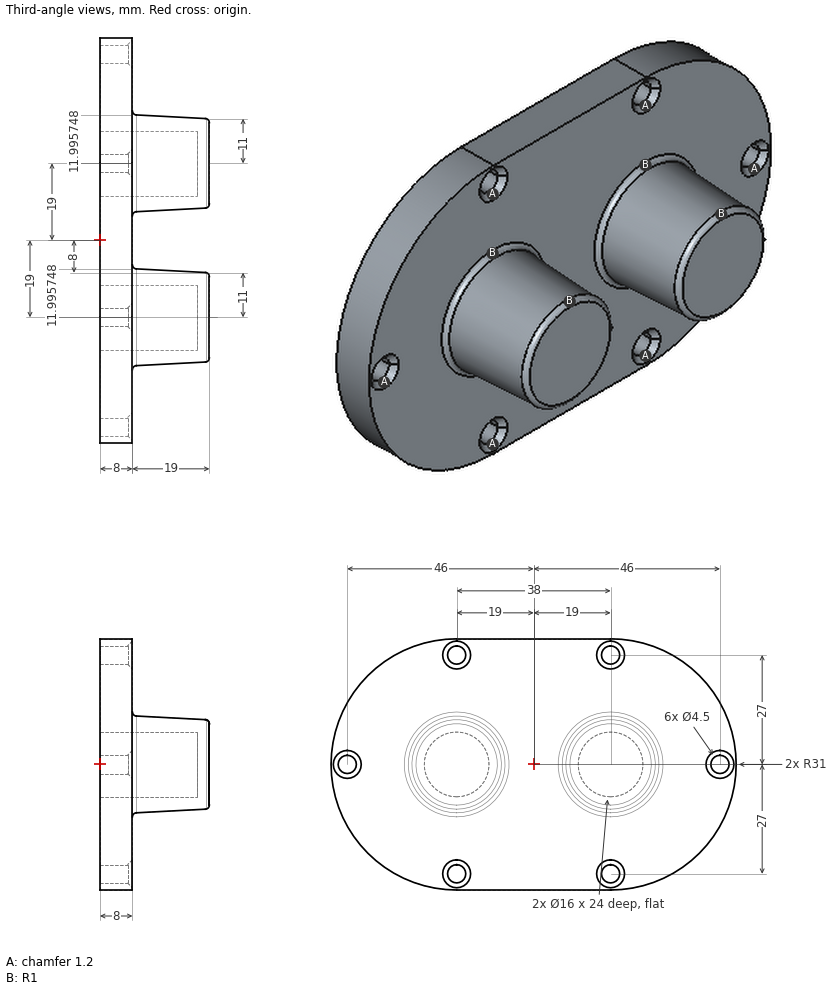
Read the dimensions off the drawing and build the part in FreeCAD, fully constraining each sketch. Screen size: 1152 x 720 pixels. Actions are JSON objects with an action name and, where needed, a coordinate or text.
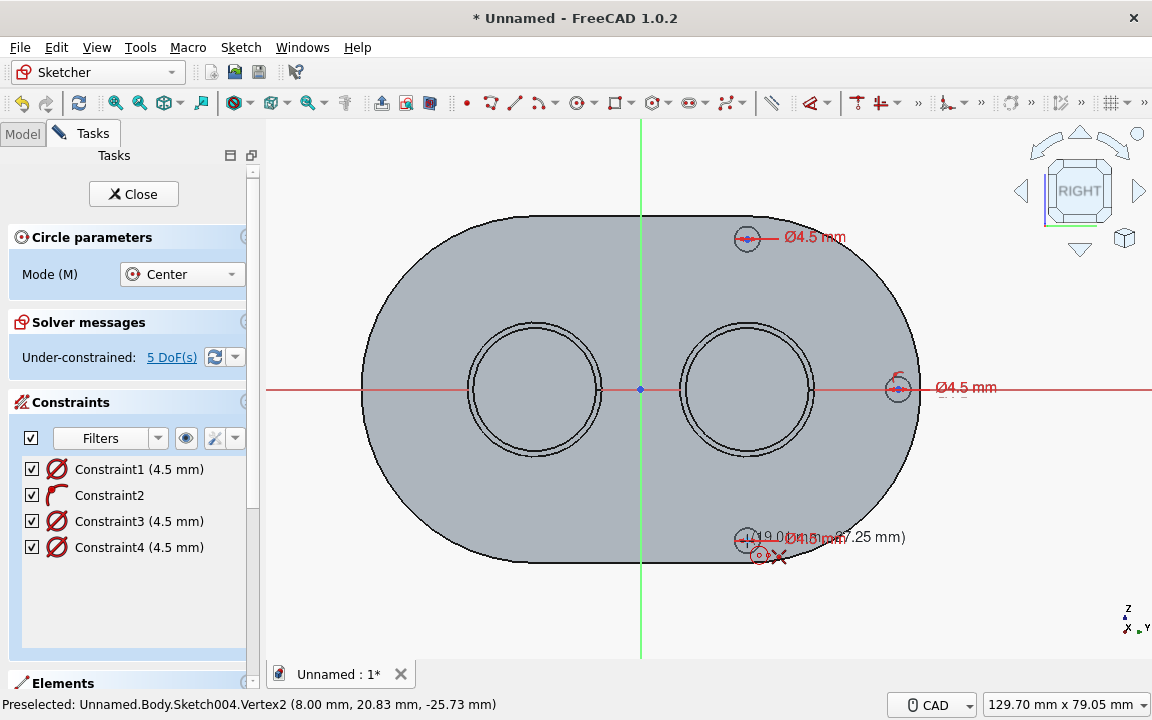
{"action": "scroll", "coordinate": [535, 239], "scroll_direction": "up", "scroll_amount": 3}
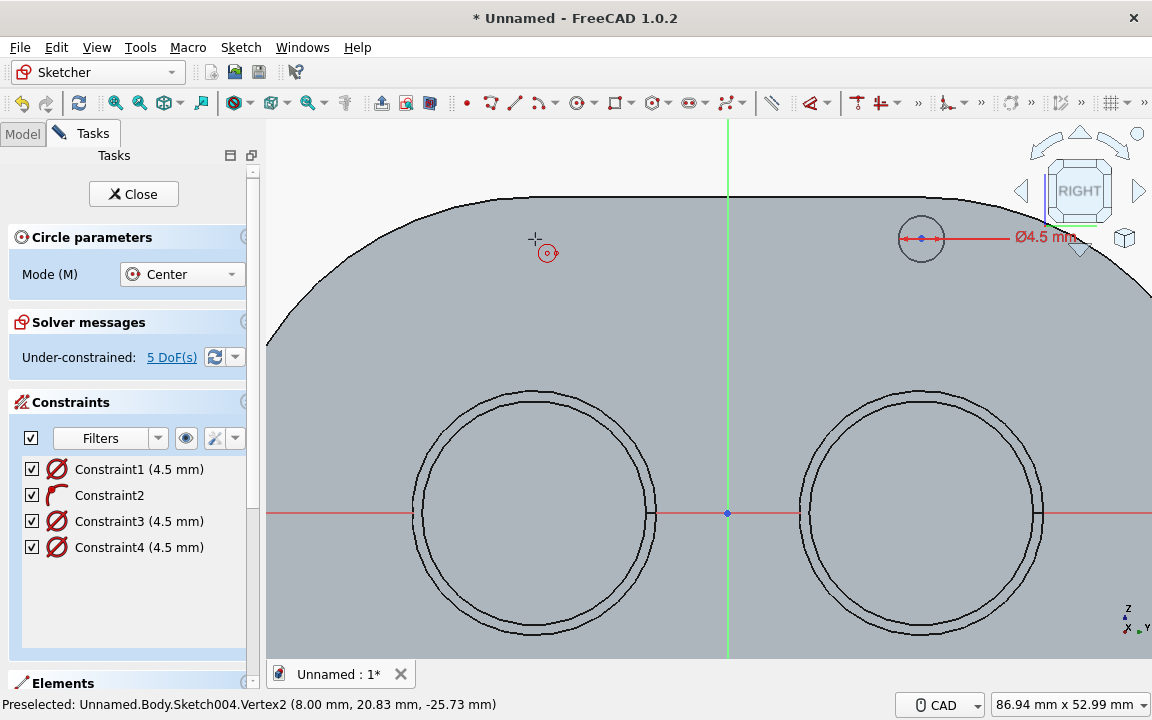
{"action": "left_click", "coordinate": [534, 238]}
{"action": "mouse_move", "coordinate": [550, 222]}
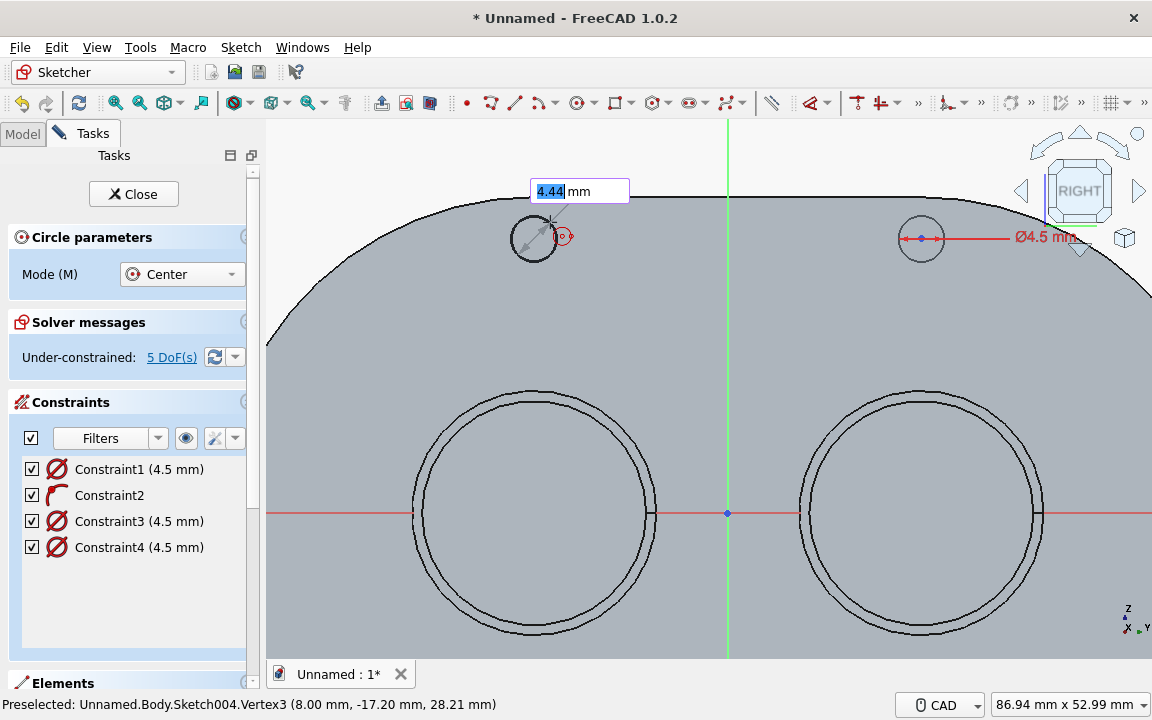
{"action": "type", "text": "4.5"}
{"action": "key", "text": "Return"}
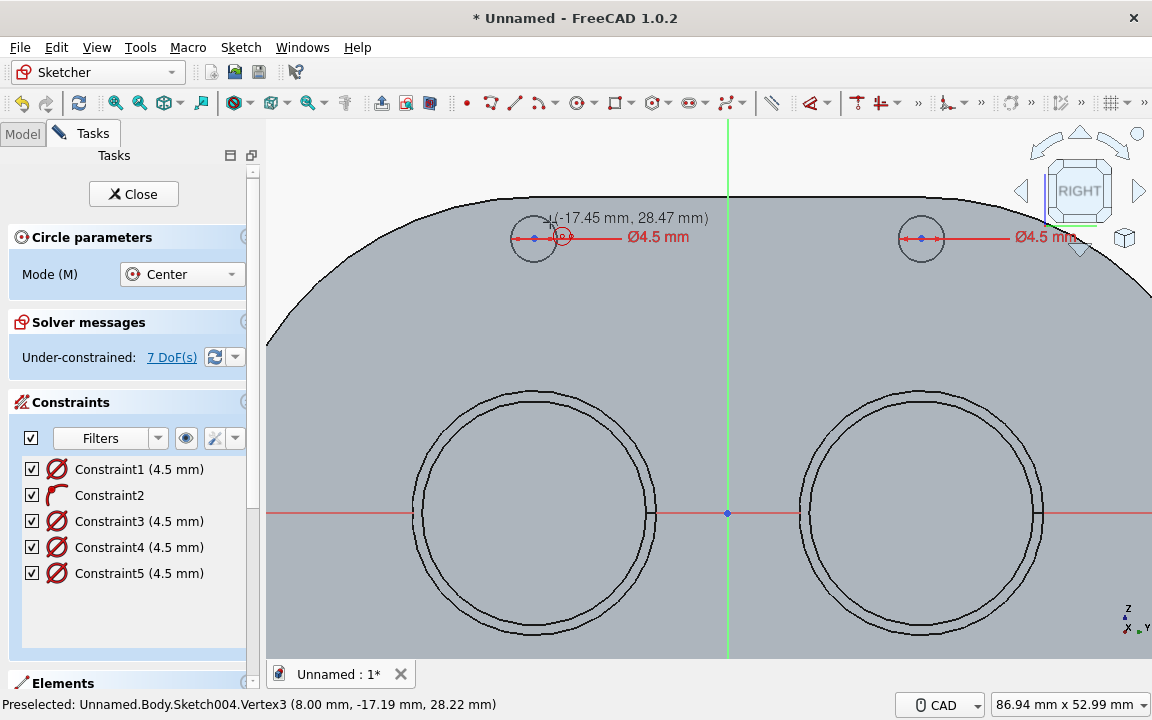
{"action": "scroll", "coordinate": [534, 238], "scroll_direction": "down", "scroll_amount": 3}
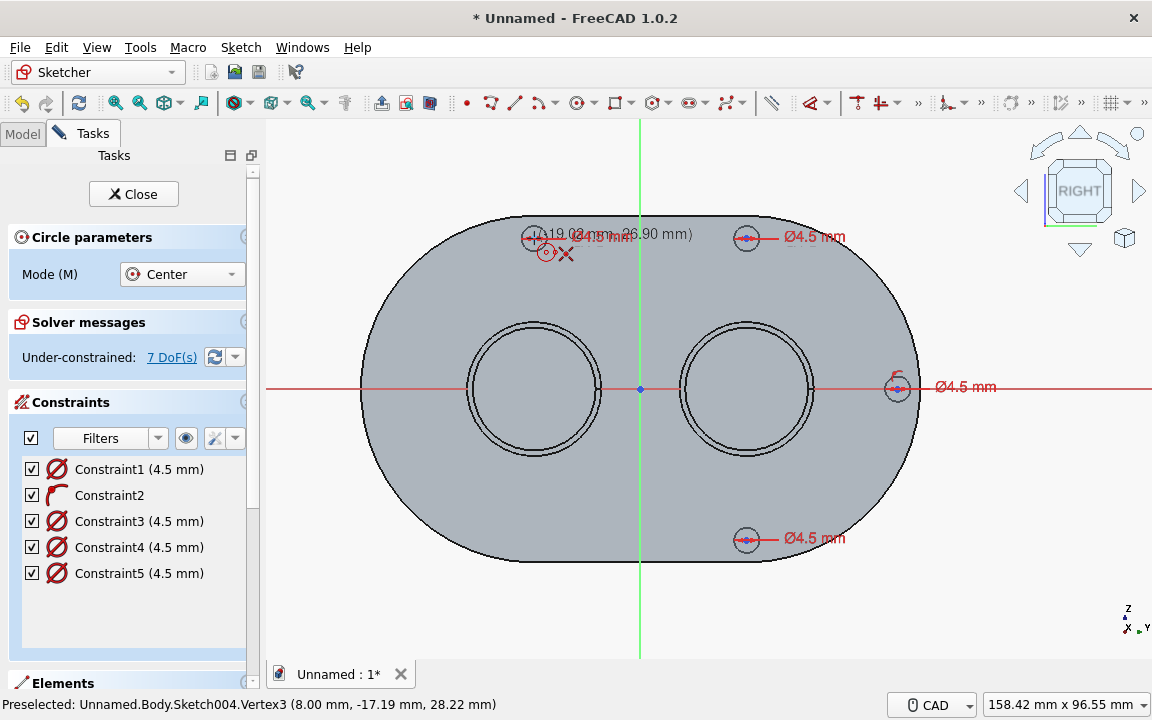
{"action": "scroll", "coordinate": [534, 540], "scroll_direction": "up", "scroll_amount": 3}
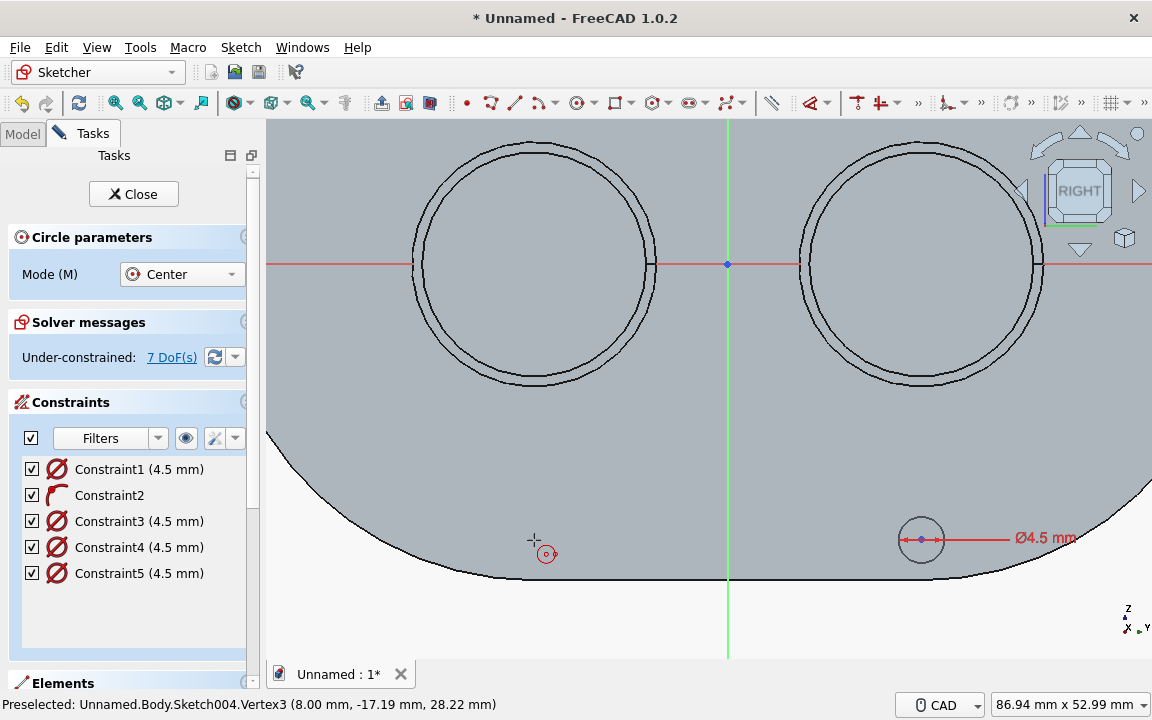
{"action": "left_click", "coordinate": [534, 539]}
{"action": "mouse_move", "coordinate": [550, 523]}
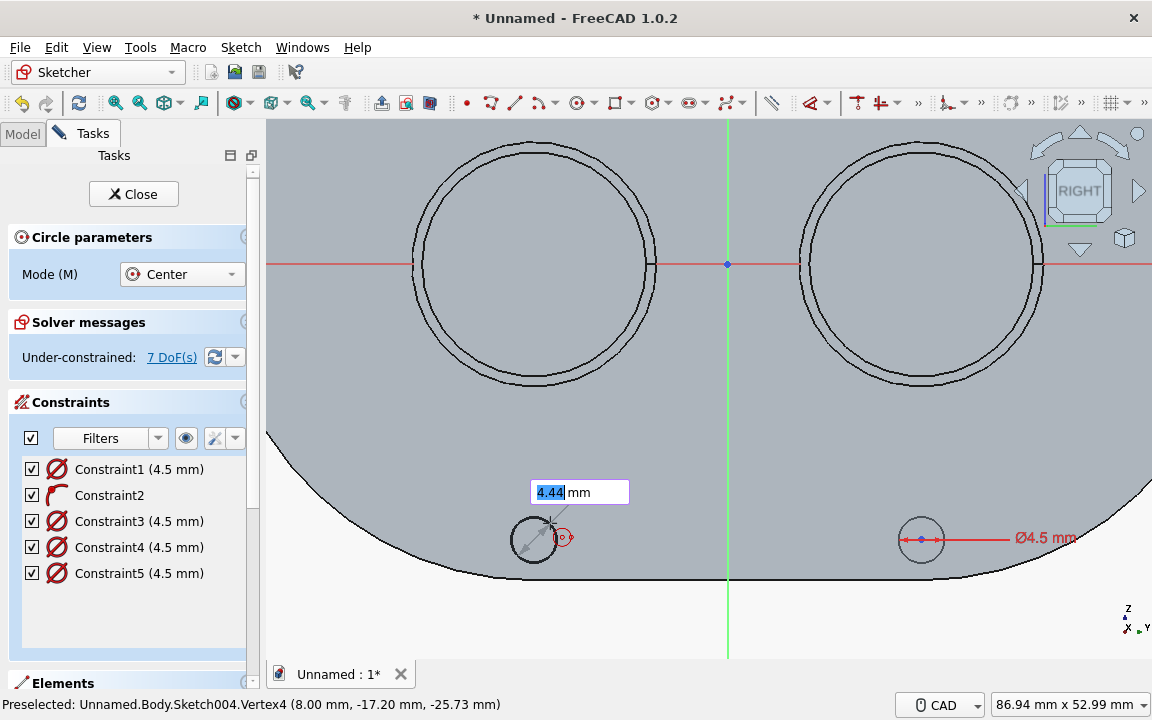
{"action": "type", "text": "4.5"}
{"action": "key", "text": "Return"}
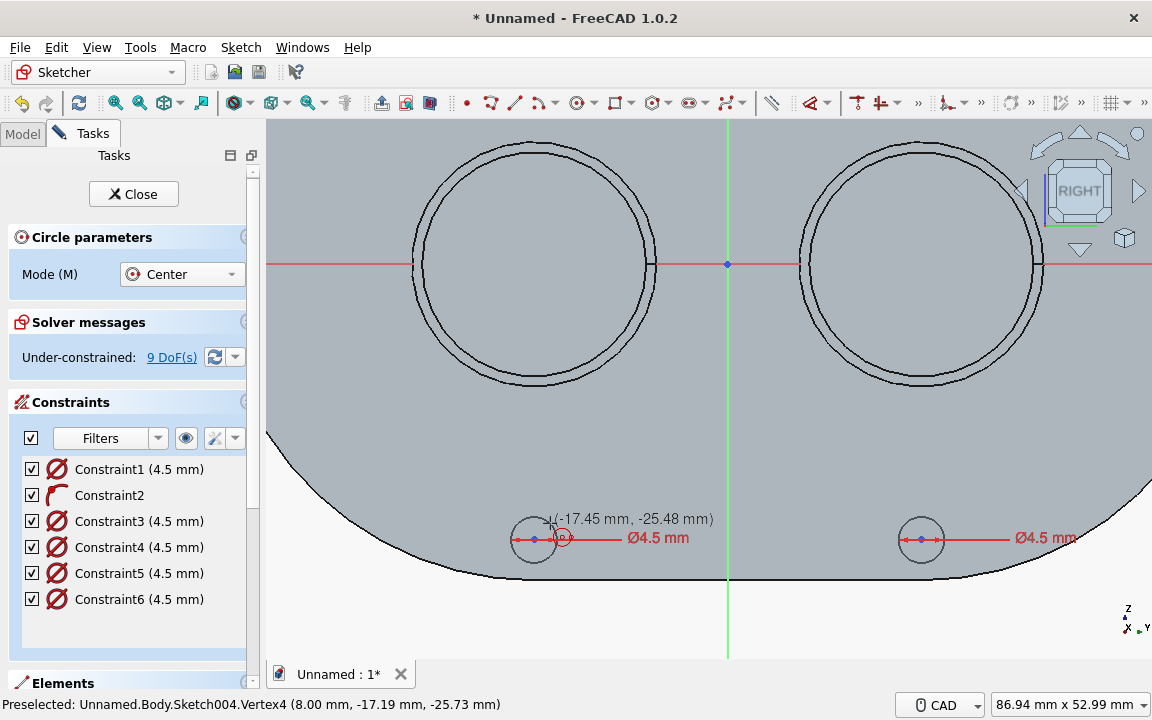
{"action": "scroll", "coordinate": [534, 541], "scroll_direction": "down", "scroll_amount": 3}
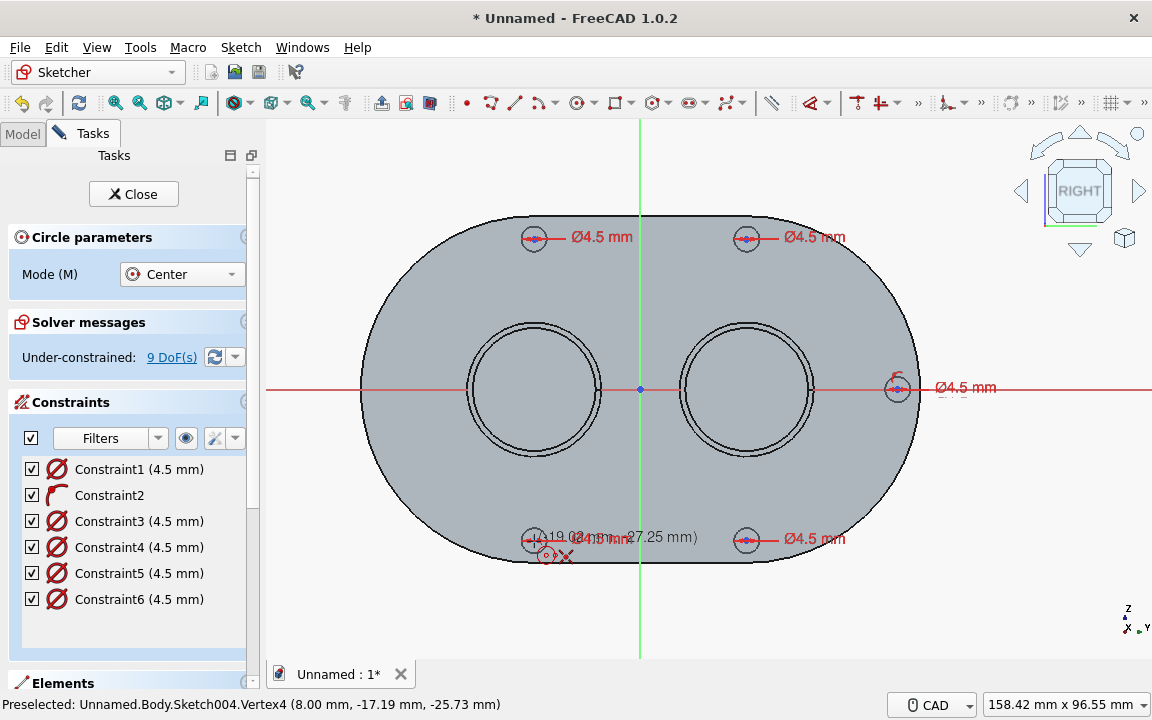
{"action": "scroll", "coordinate": [383, 390], "scroll_direction": "up", "scroll_amount": 3}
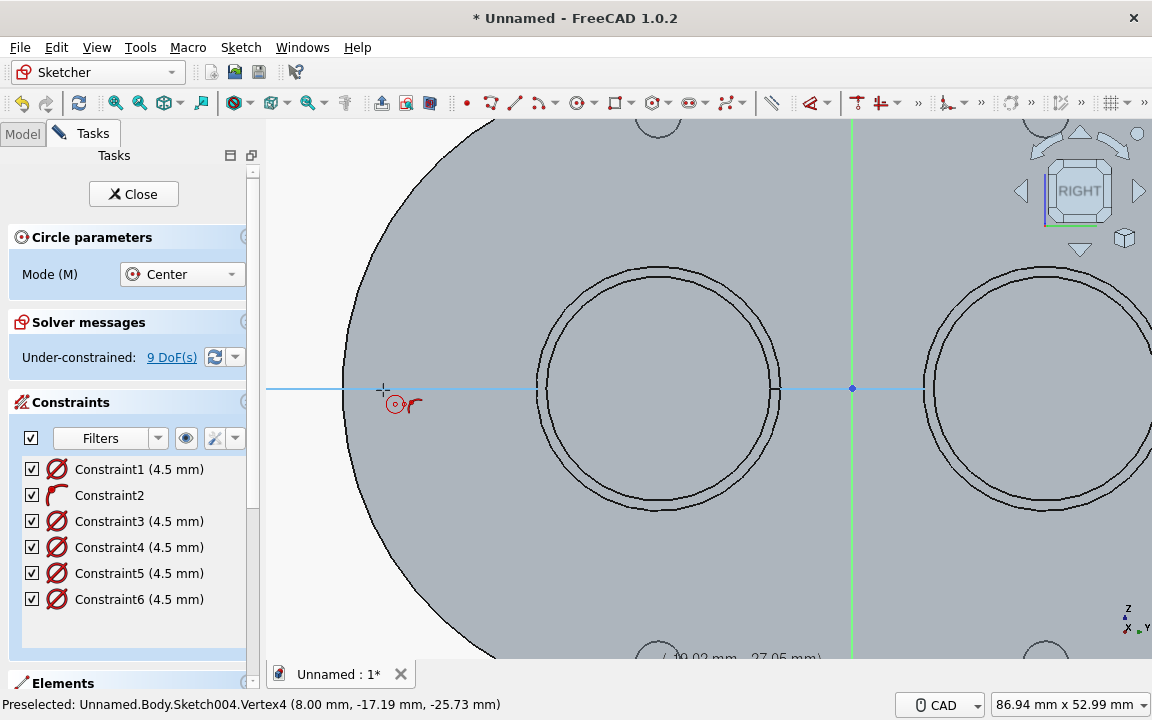
{"action": "left_click", "coordinate": [383, 389]}
{"action": "mouse_move", "coordinate": [400, 373]}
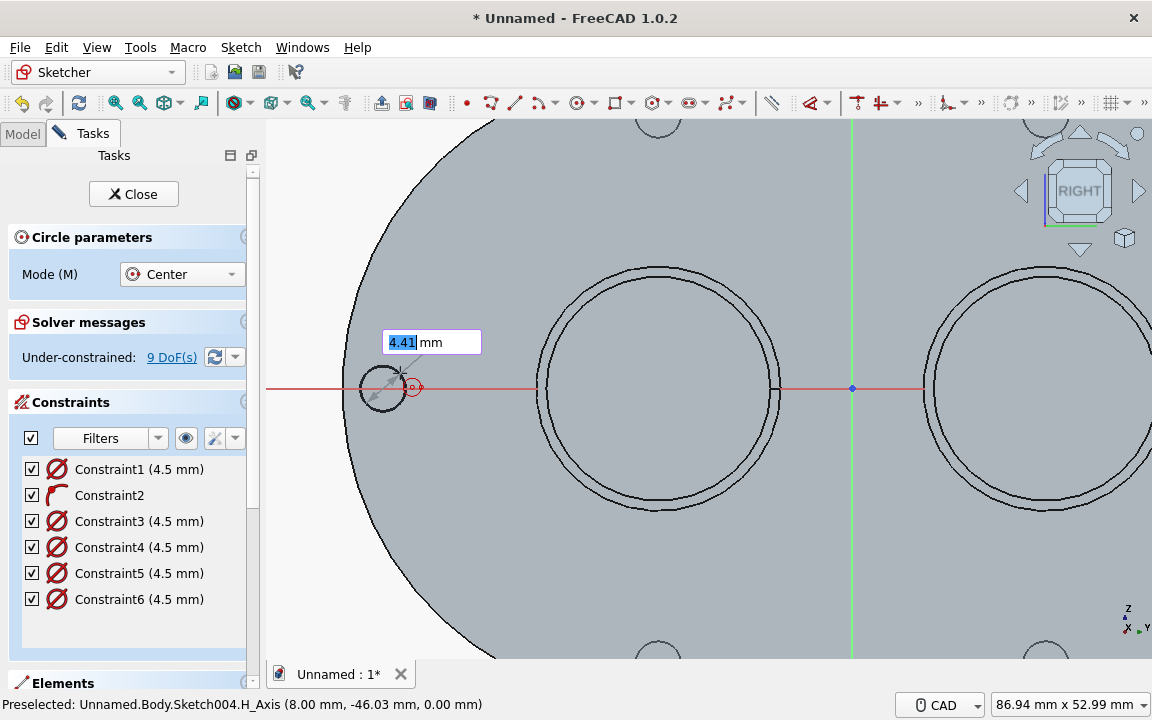
{"action": "type", "text": "4.5"}
{"action": "key", "text": "Return"}
{"action": "key", "text": "Escape"}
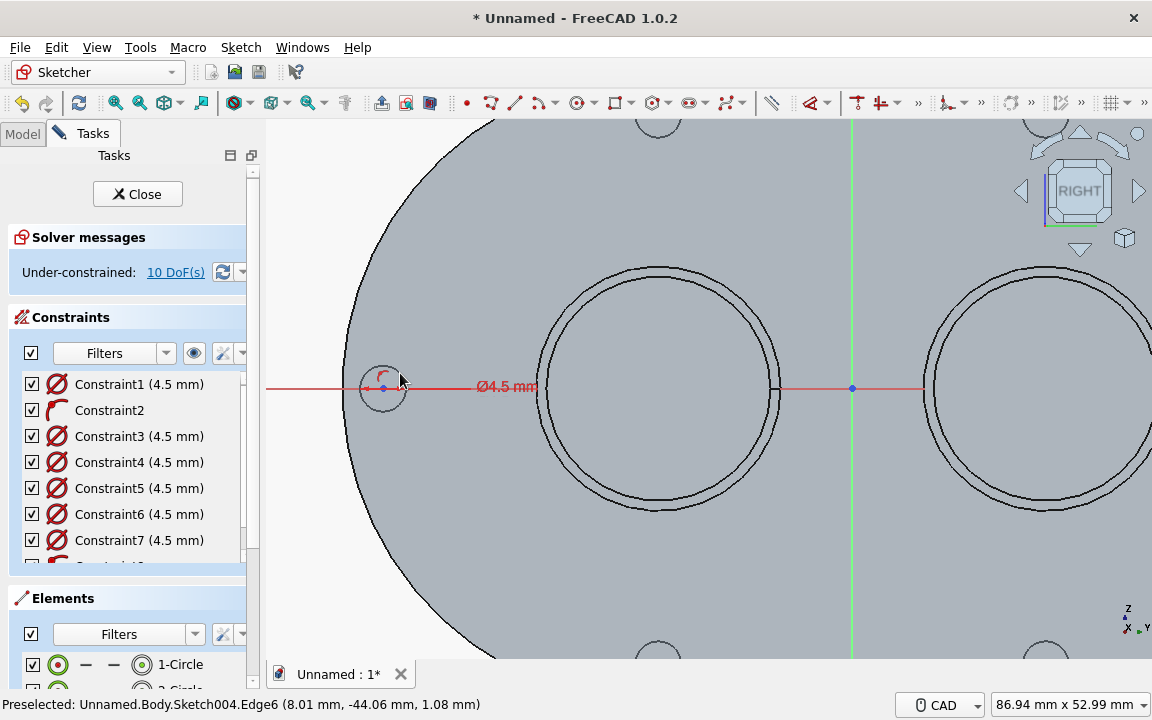
{"action": "left_click", "coordinate": [810, 104]}